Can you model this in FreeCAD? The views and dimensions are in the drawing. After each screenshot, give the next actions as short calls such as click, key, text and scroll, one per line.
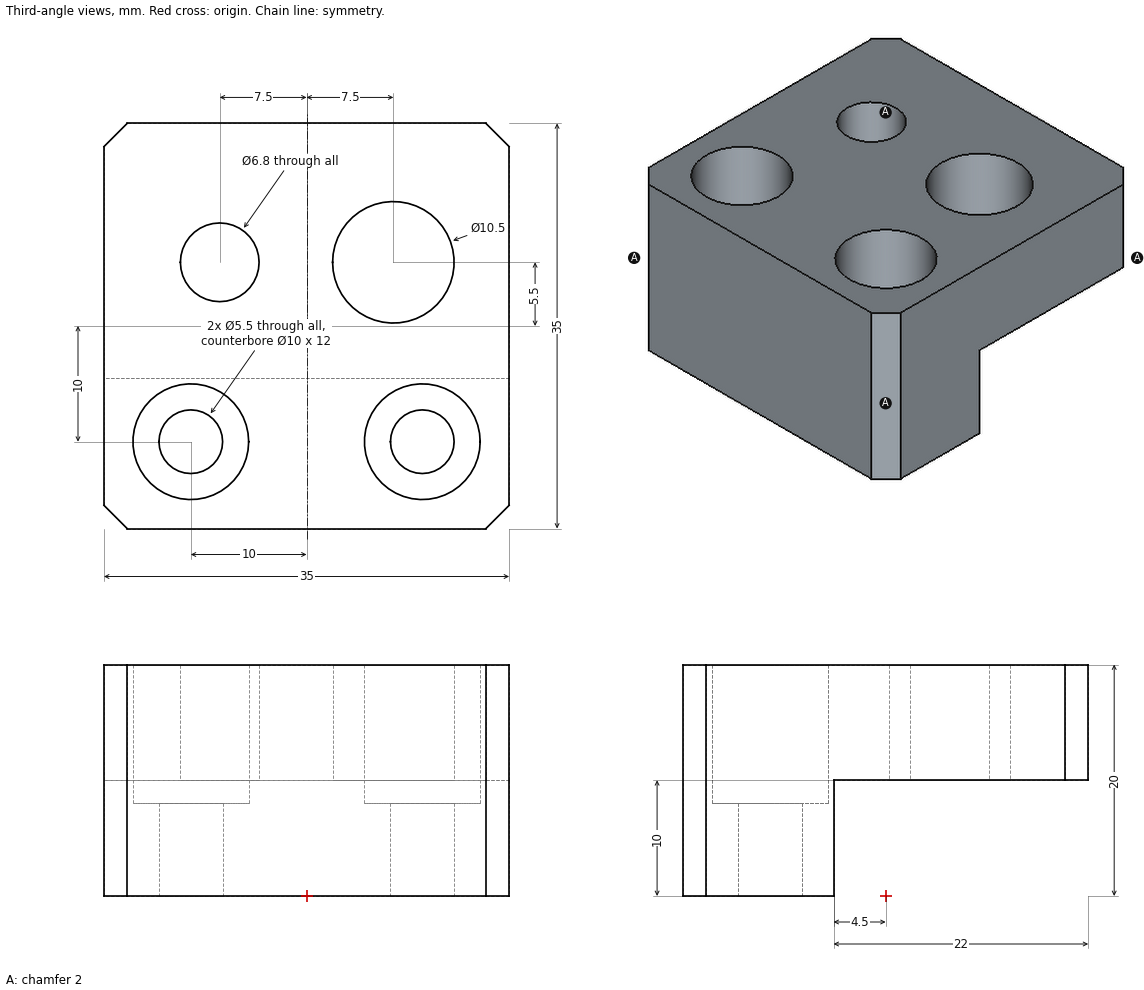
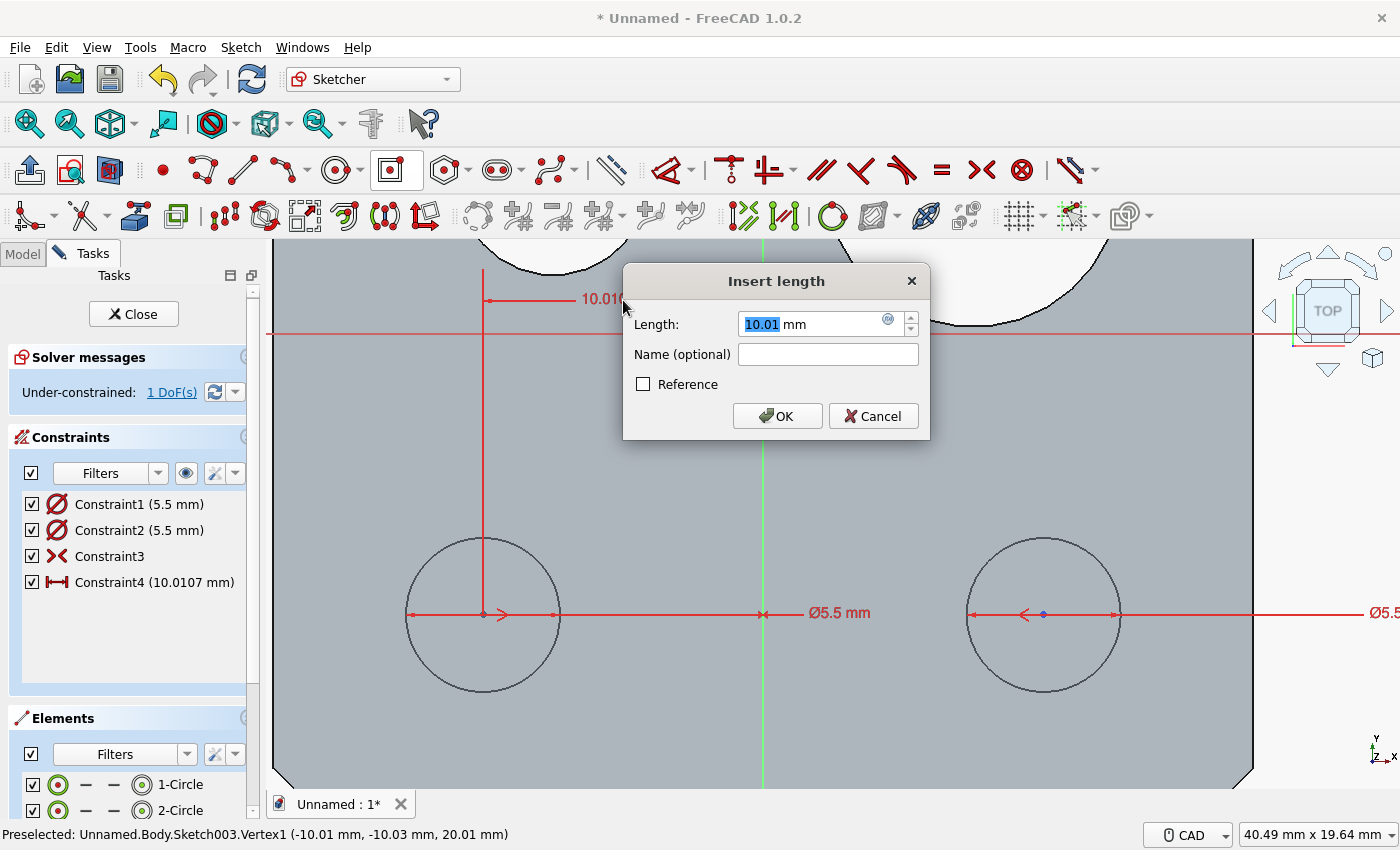
text(10)
key(Return)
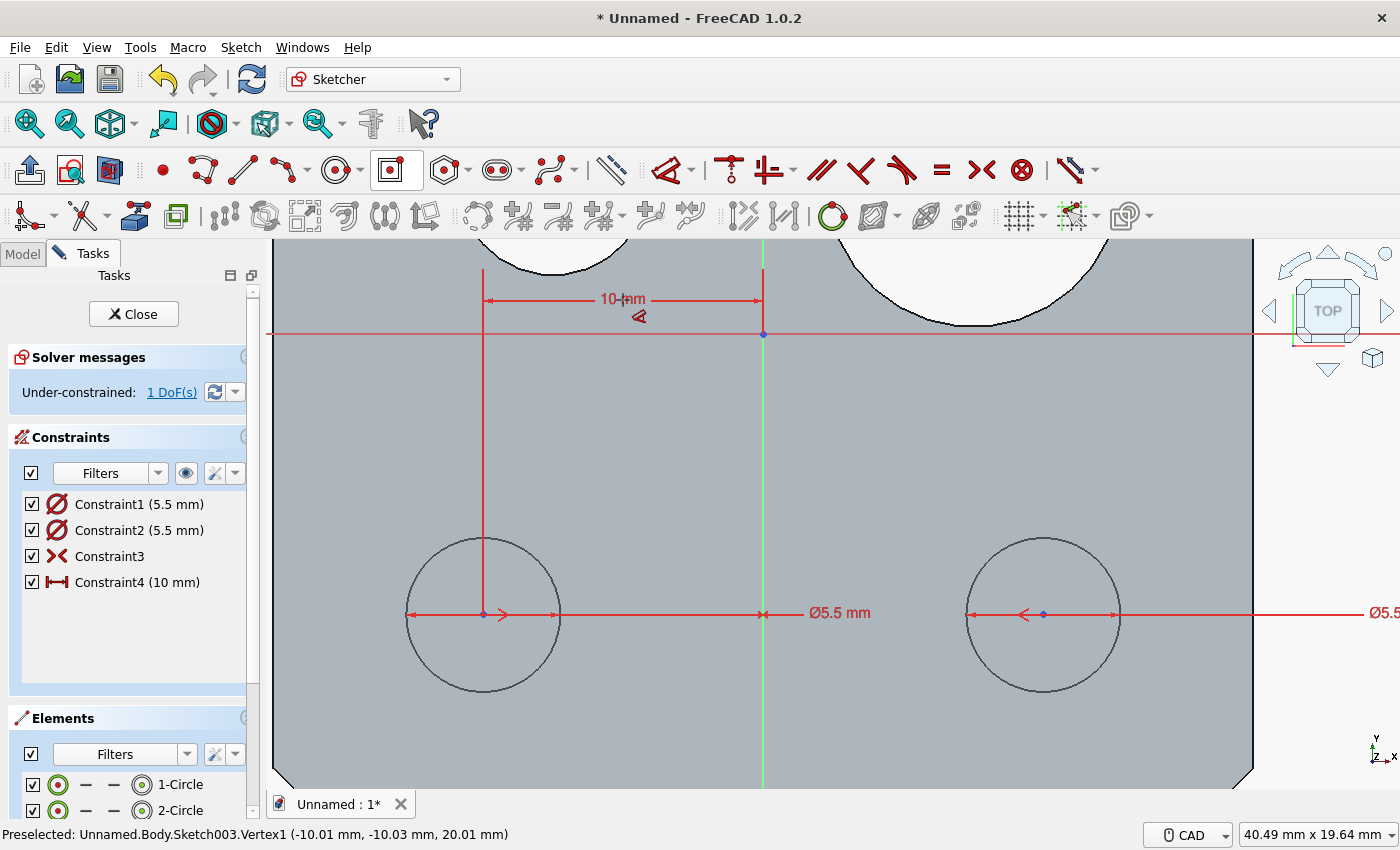
click(483, 615)
click(449, 475)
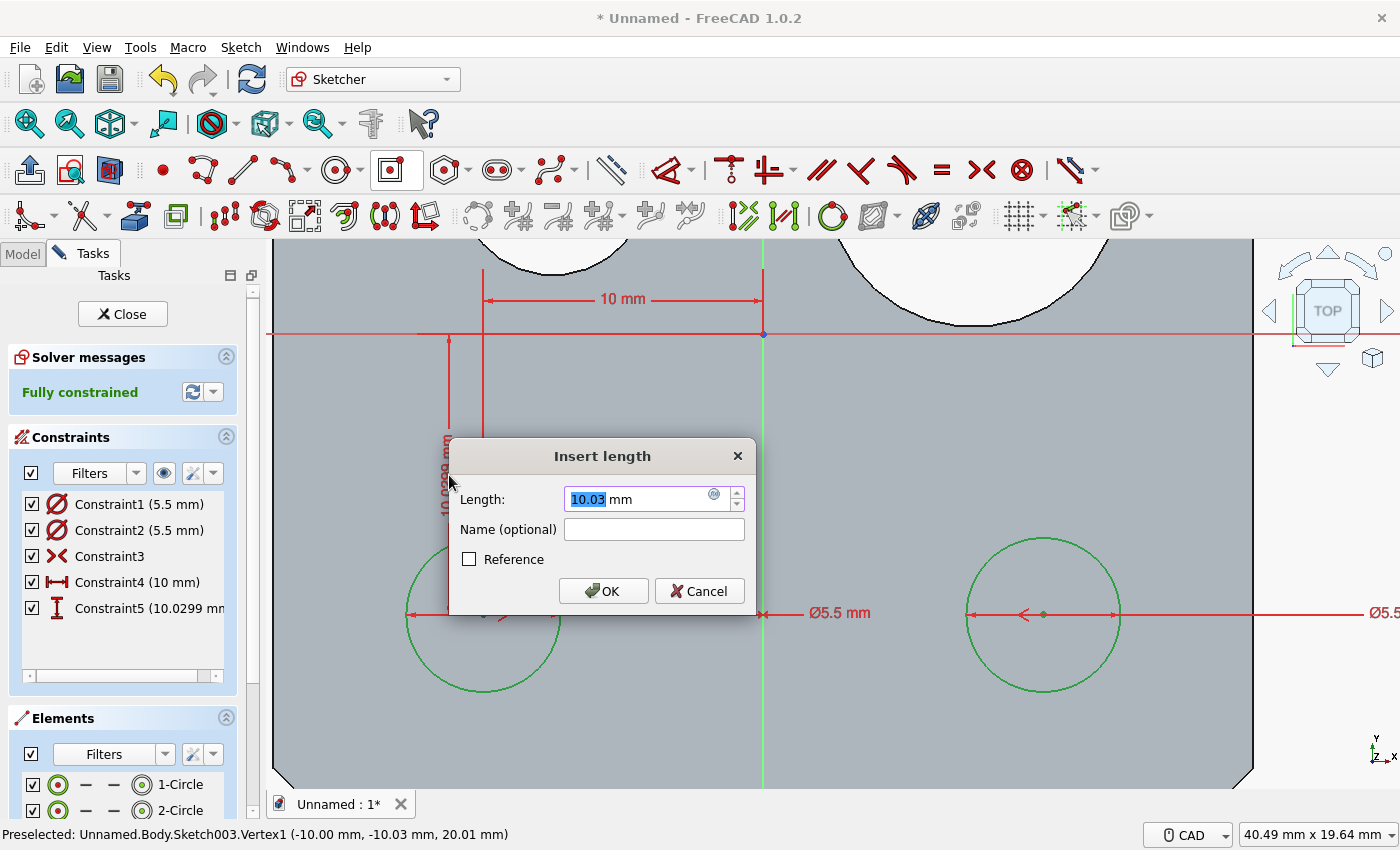
text(10)
key(Return)
key(Escape)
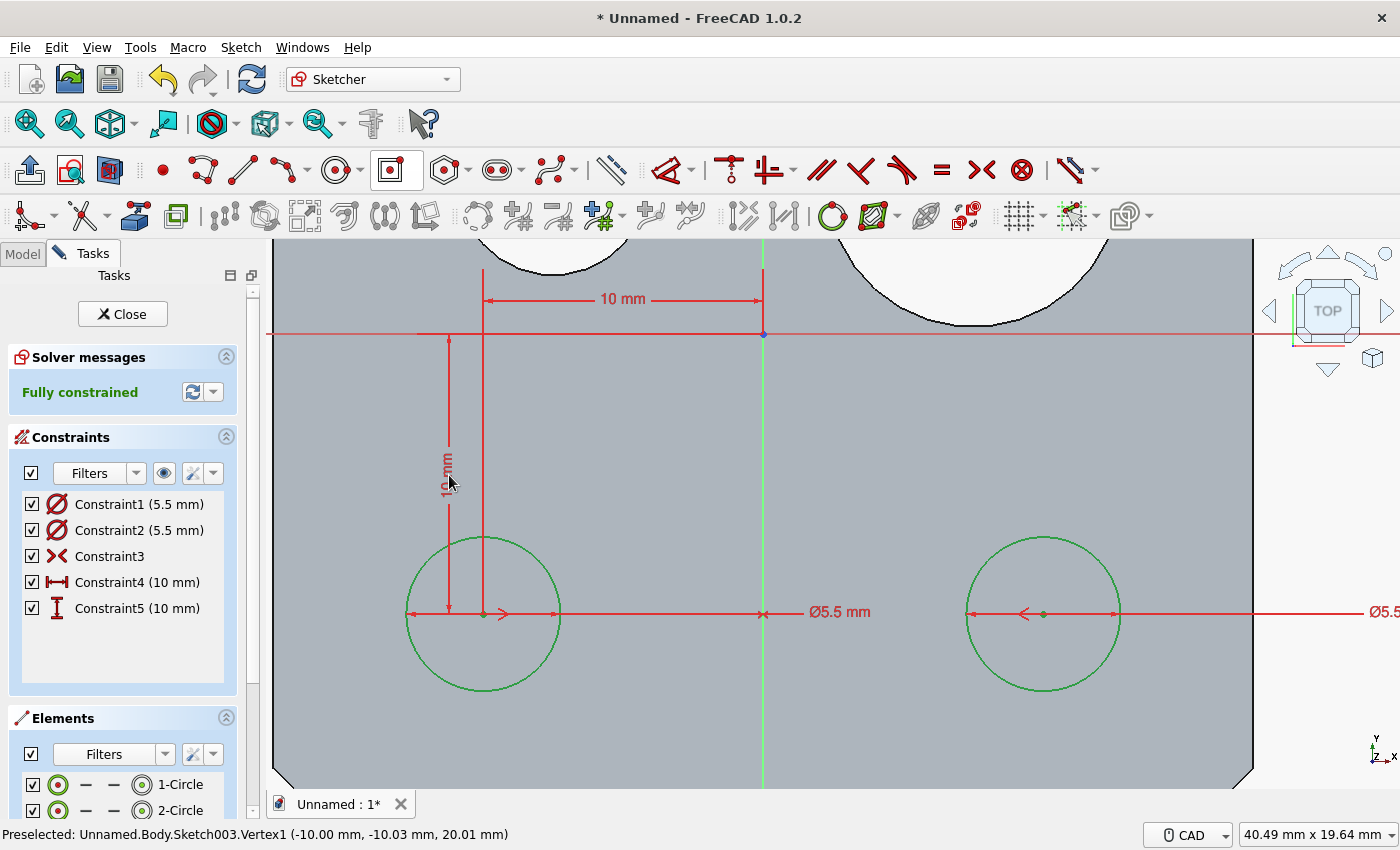
click(123, 314)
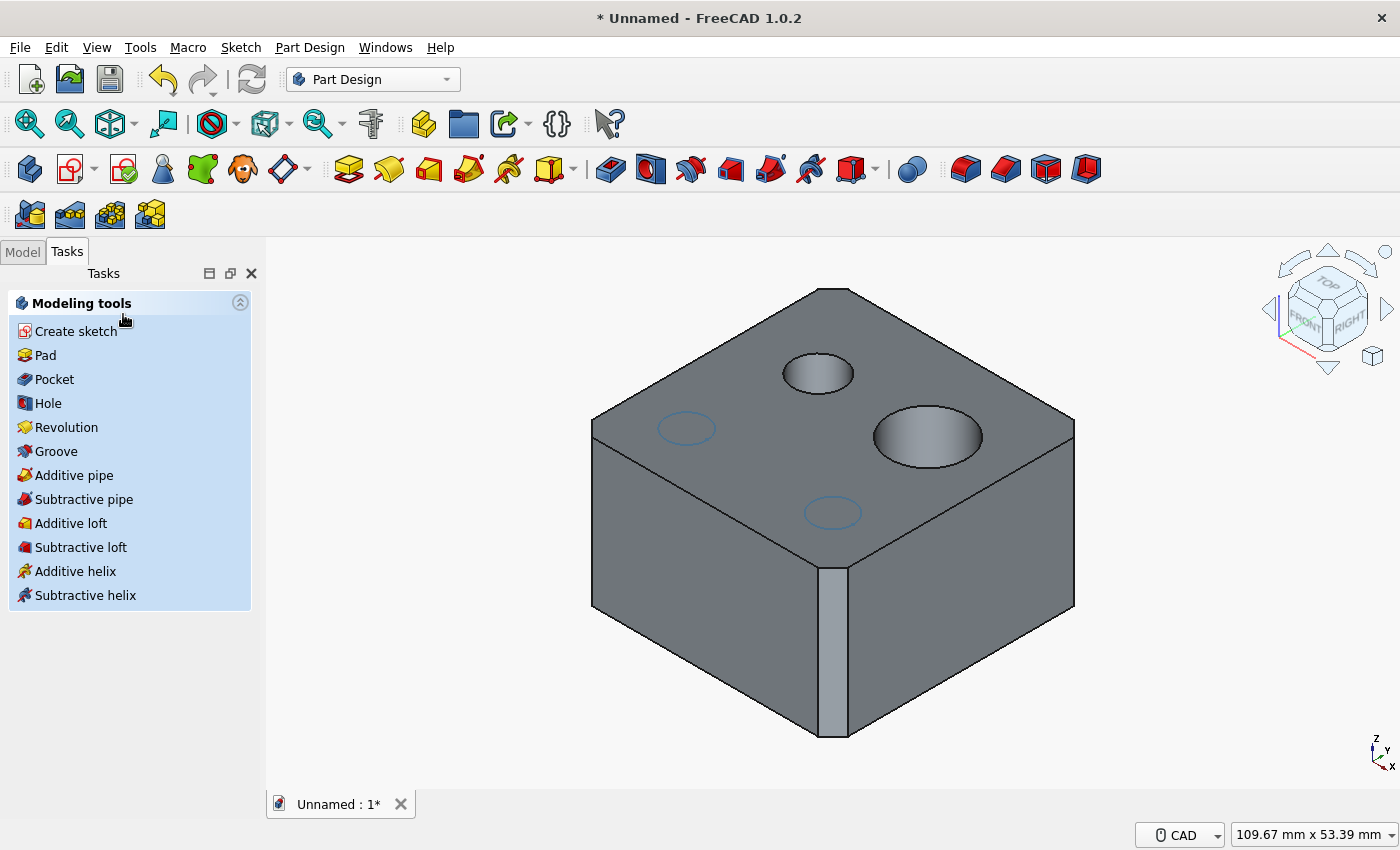
click(652, 170)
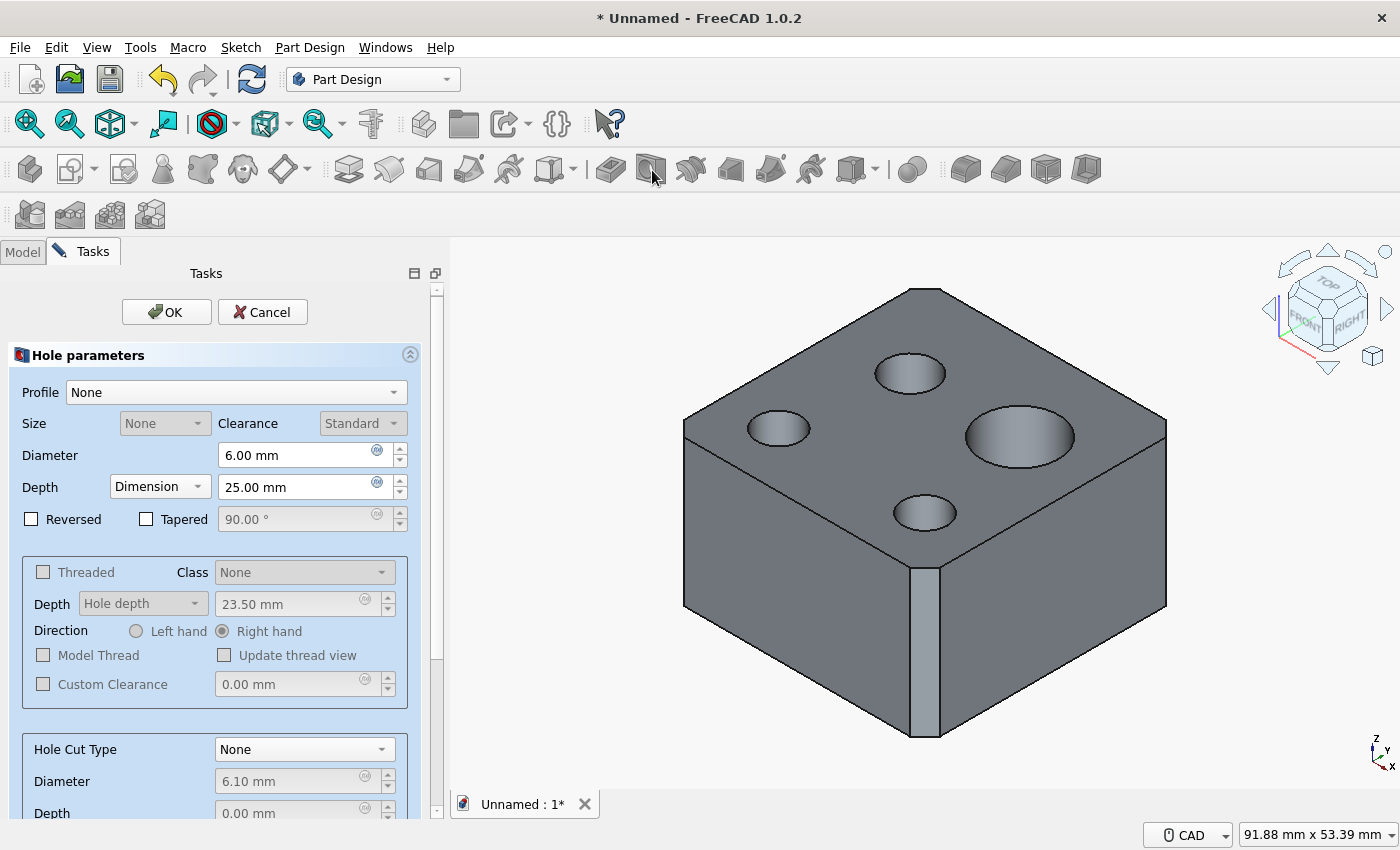
triple_click(305, 455)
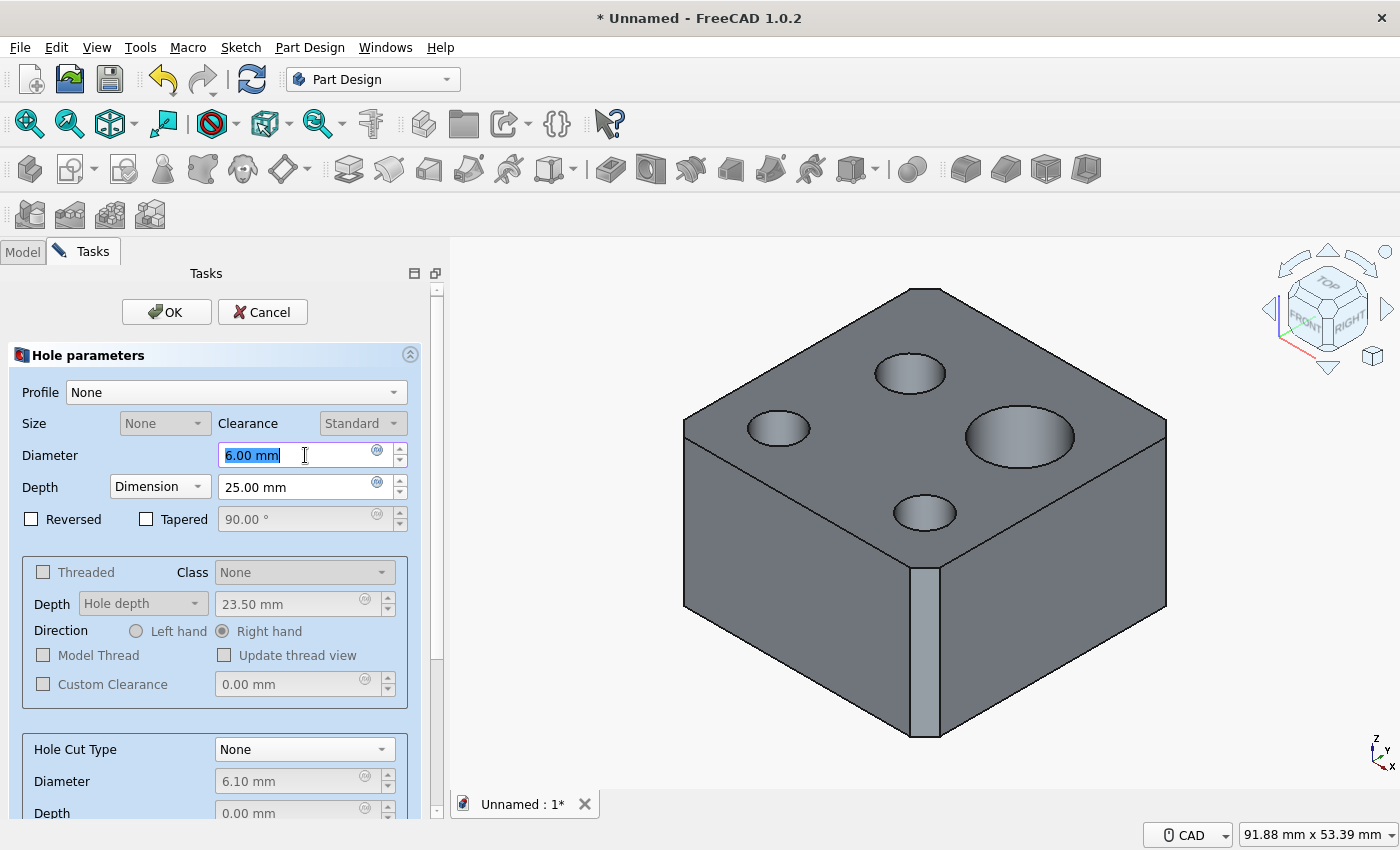
text(5.5)
key(Tab)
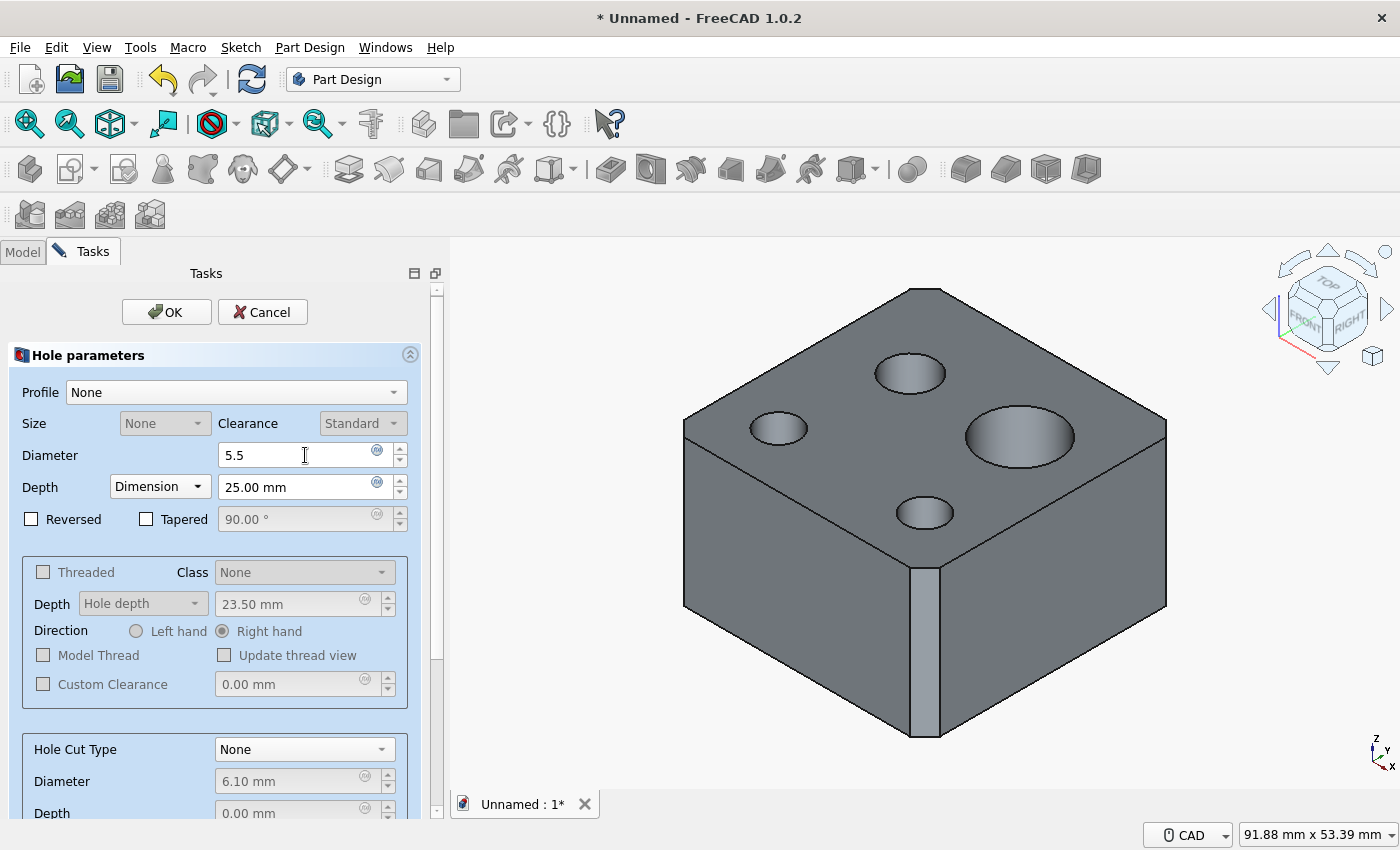
click(161, 486)